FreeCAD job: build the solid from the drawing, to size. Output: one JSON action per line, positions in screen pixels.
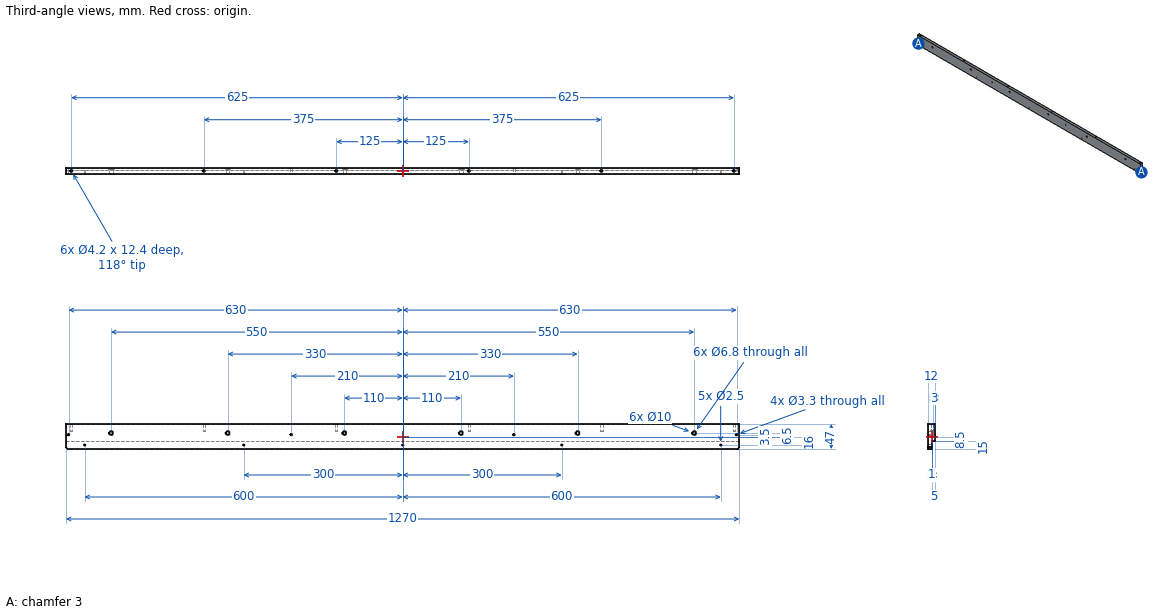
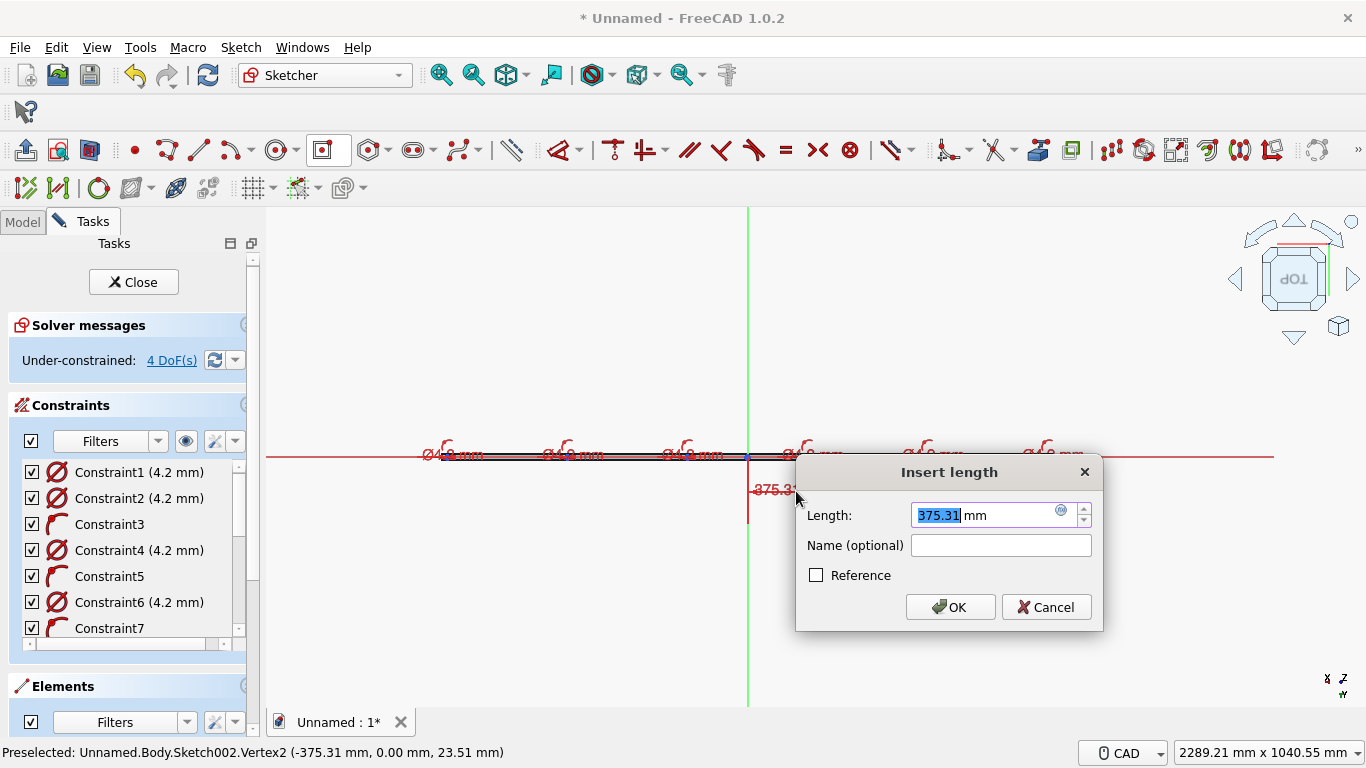
{"action": "type", "text": "375"}
{"action": "key", "text": "Return"}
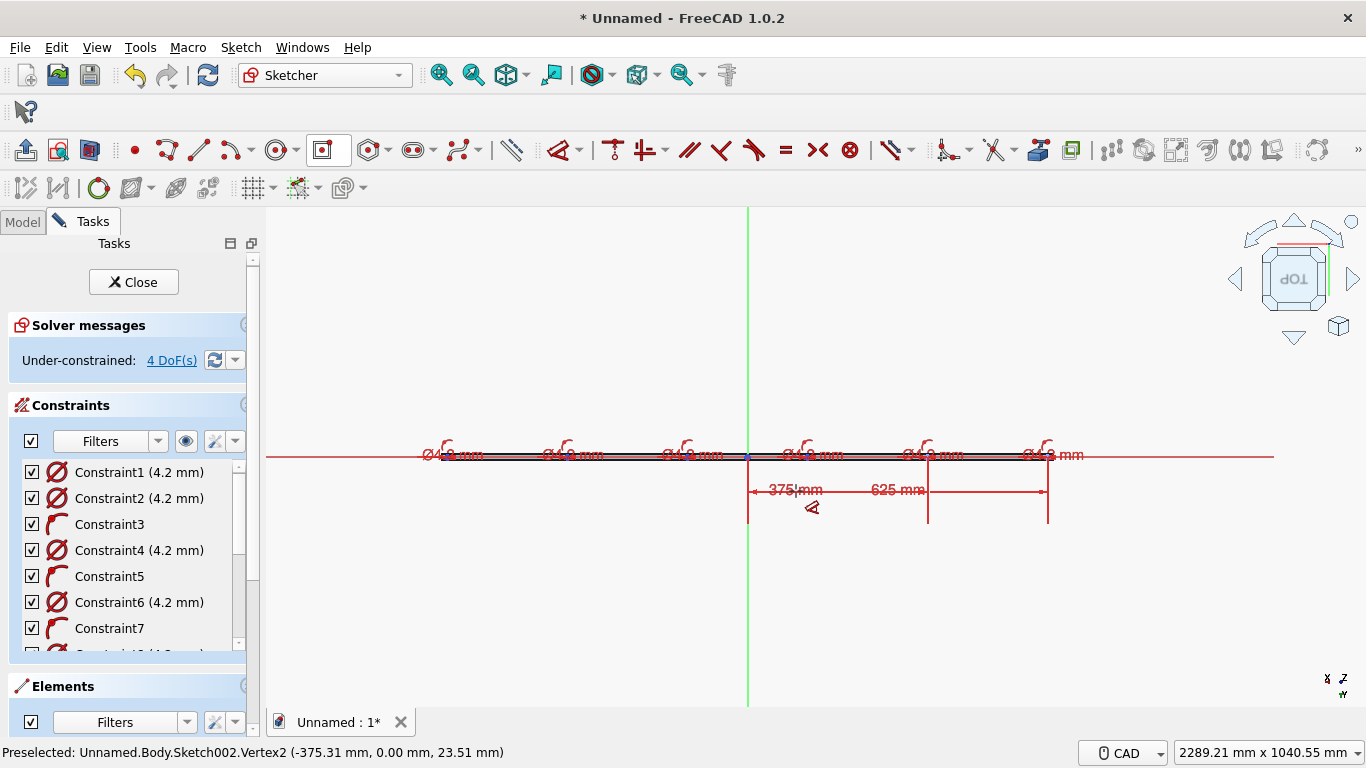
{"action": "left_click", "coordinate": [808, 457]}
{"action": "left_click", "coordinate": [778, 423]}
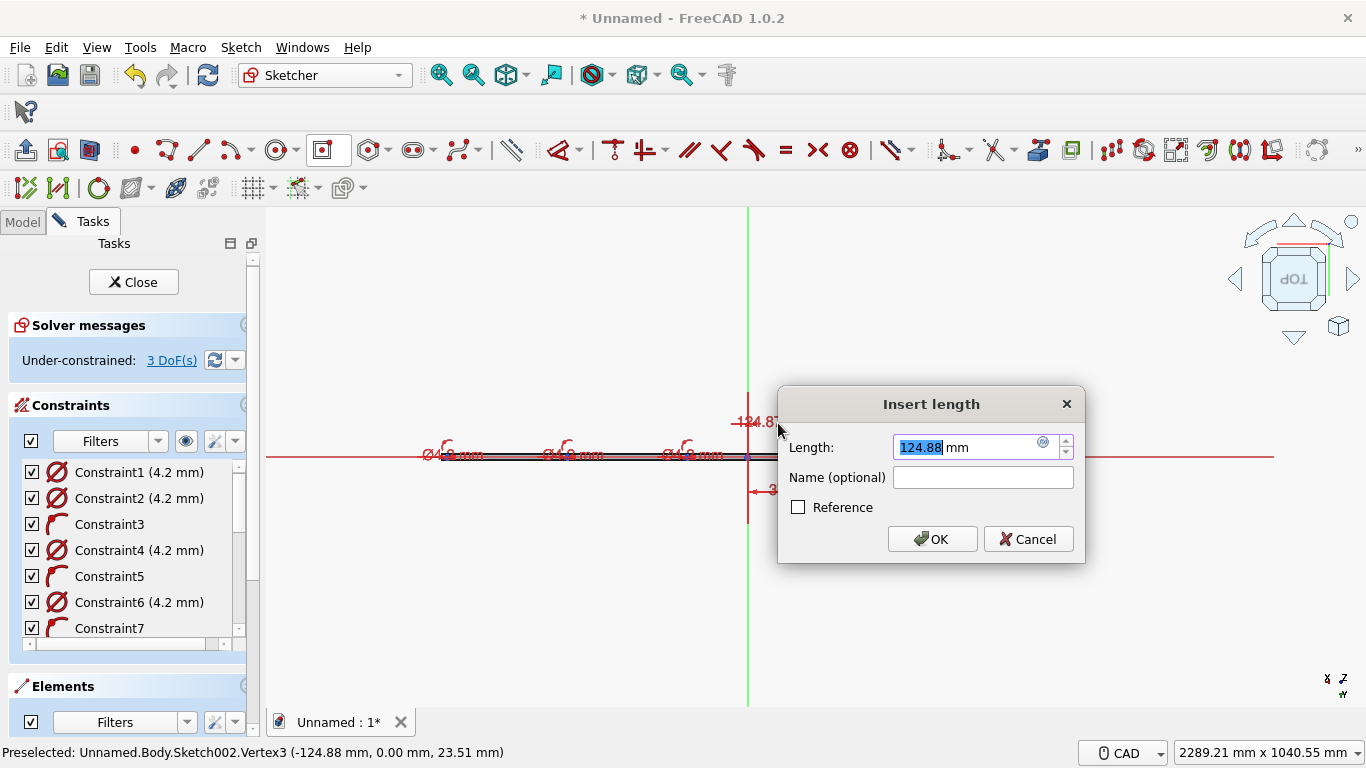
{"action": "type", "text": "125"}
{"action": "key", "text": "Return"}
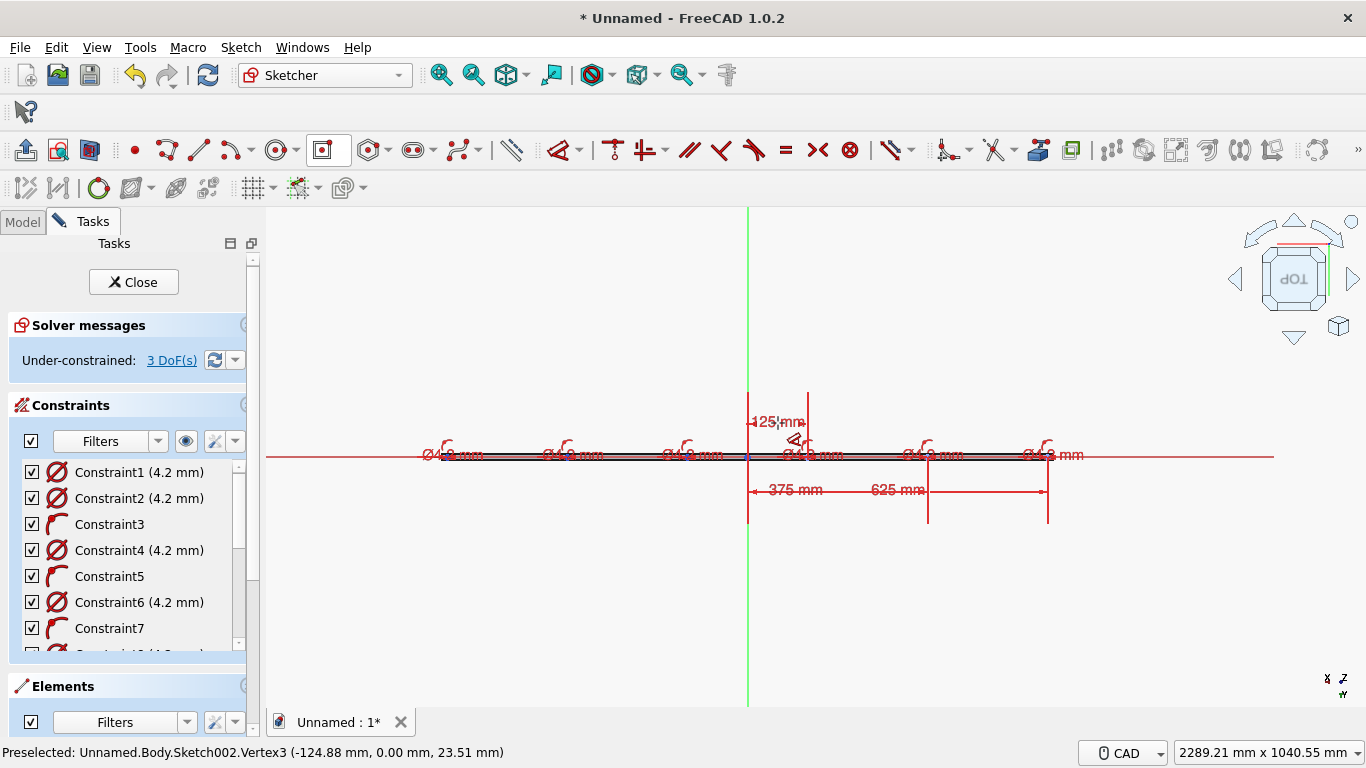
{"action": "left_click", "coordinate": [687, 457]}
{"action": "left_click", "coordinate": [717, 491]}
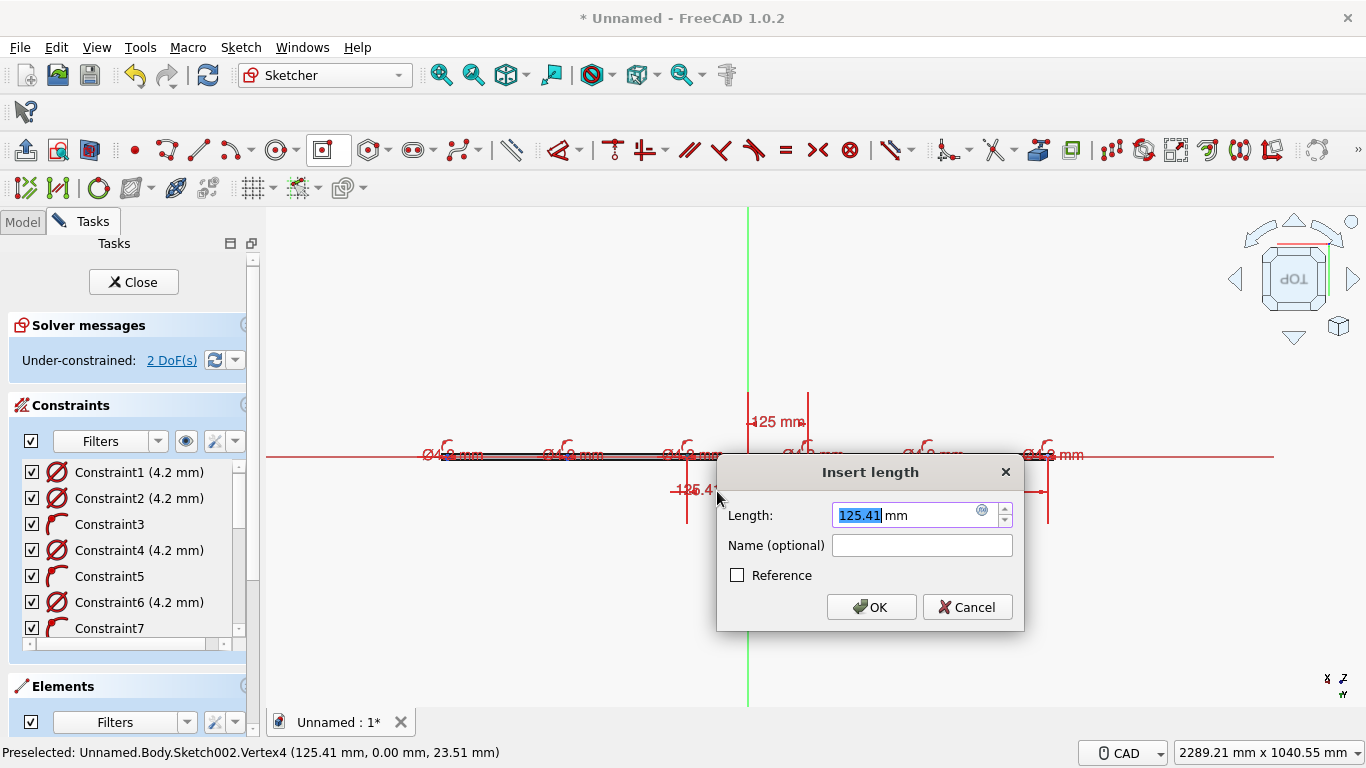
{"action": "type", "text": "125"}
{"action": "key", "text": "Return"}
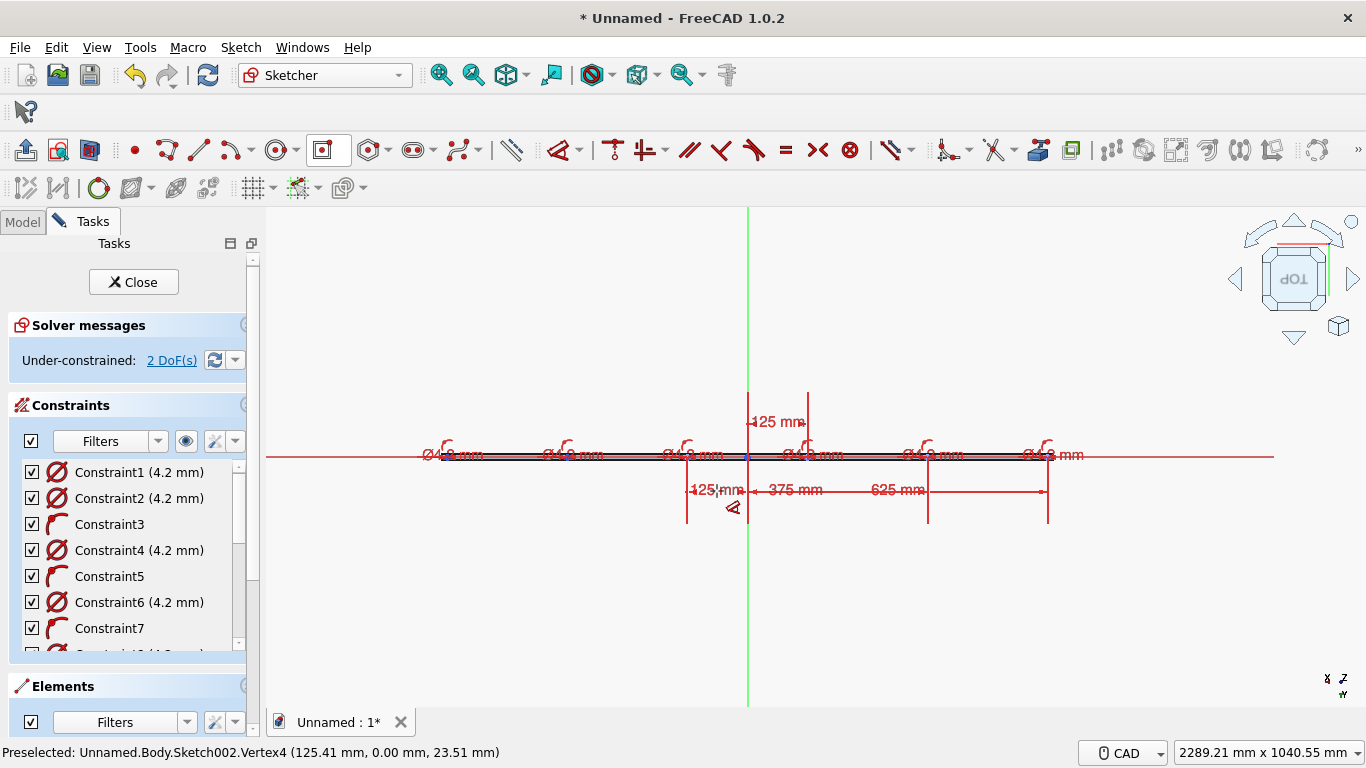
{"action": "left_click", "coordinate": [568, 457]}
{"action": "left_click", "coordinate": [616, 491]}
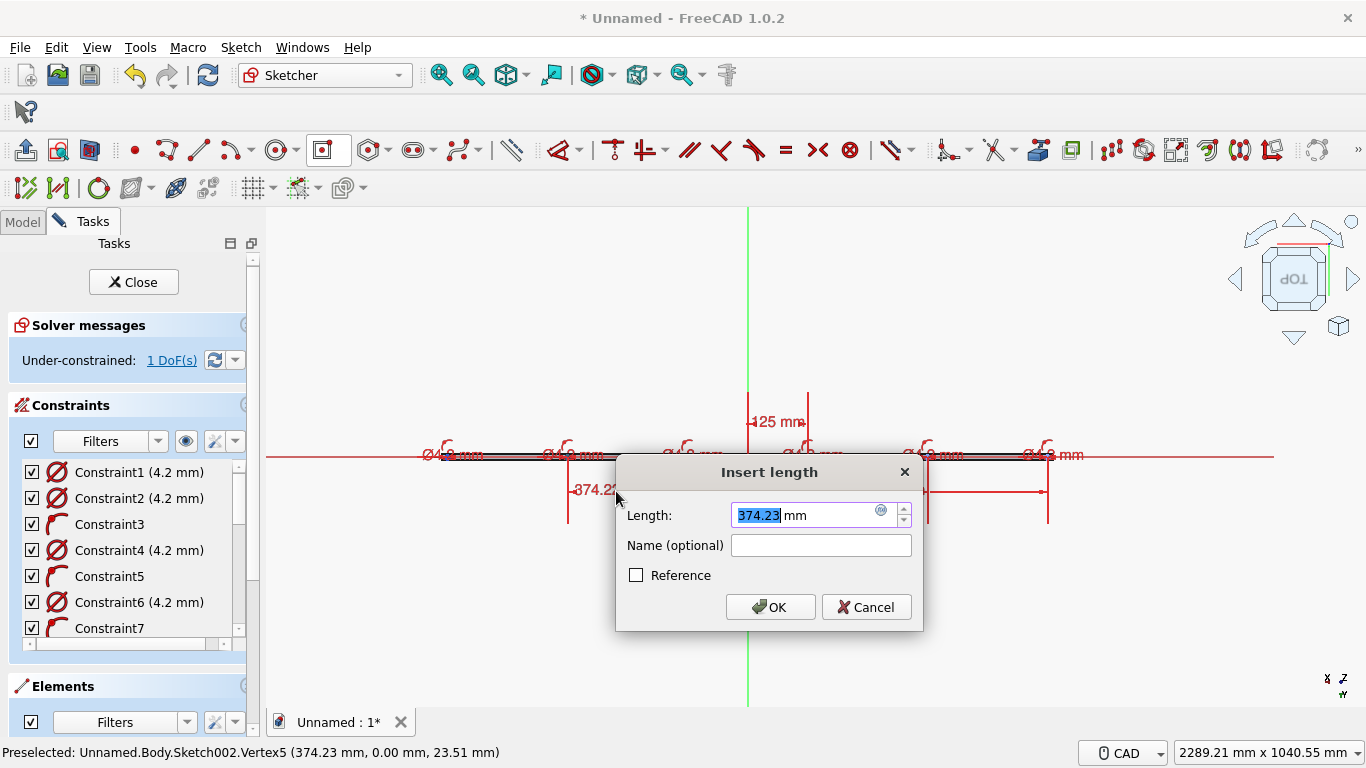
{"action": "type", "text": "375"}
{"action": "key", "text": "Return"}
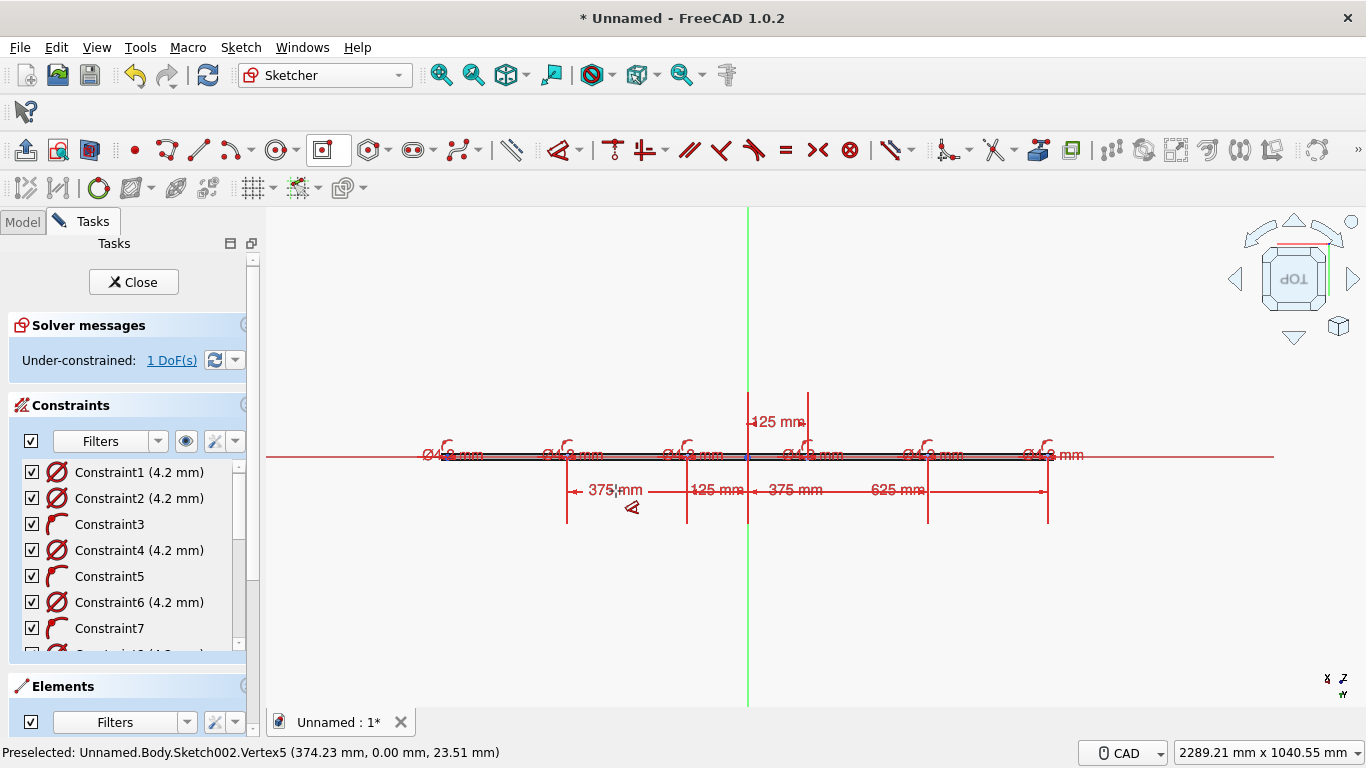
{"action": "left_click", "coordinate": [447, 457]}
{"action": "left_click", "coordinate": [528, 491]}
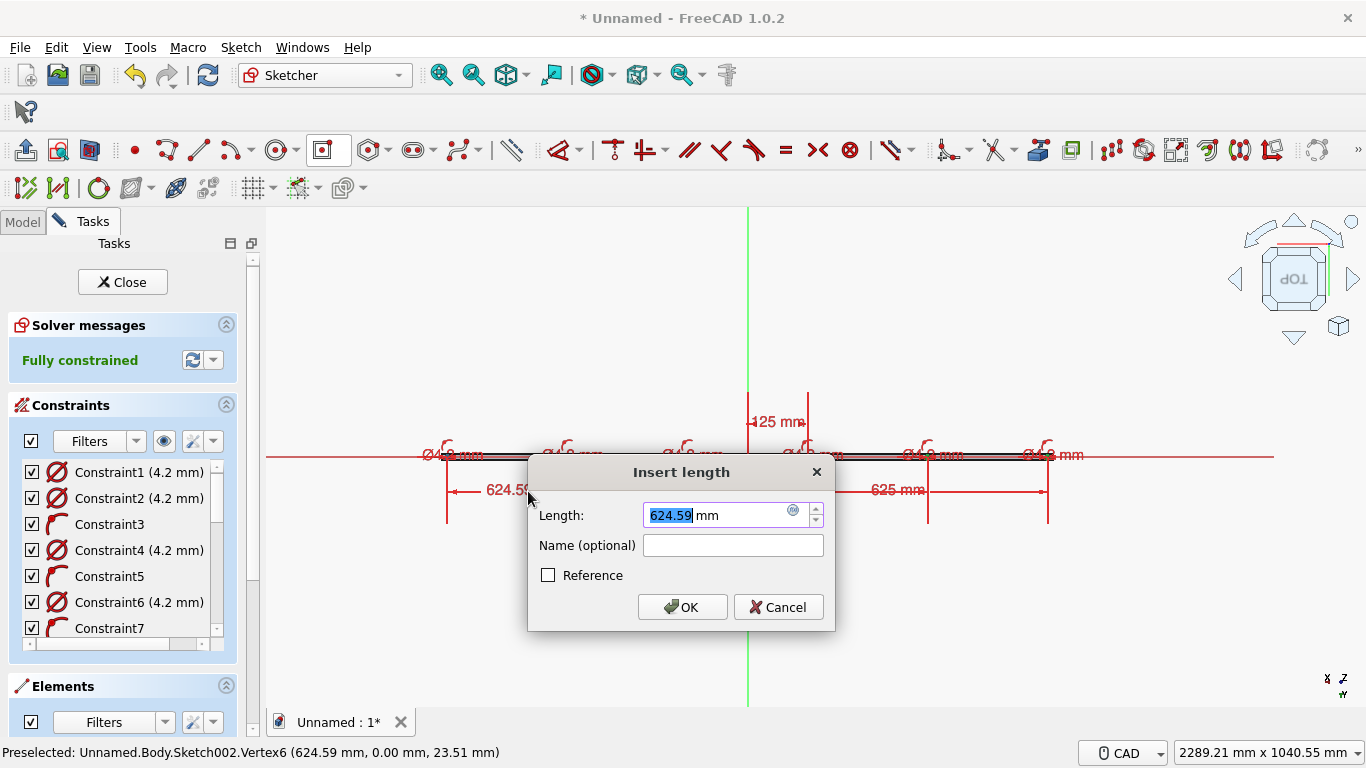
{"action": "type", "text": "625"}
{"action": "key", "text": "Return"}
{"action": "key", "text": "Escape"}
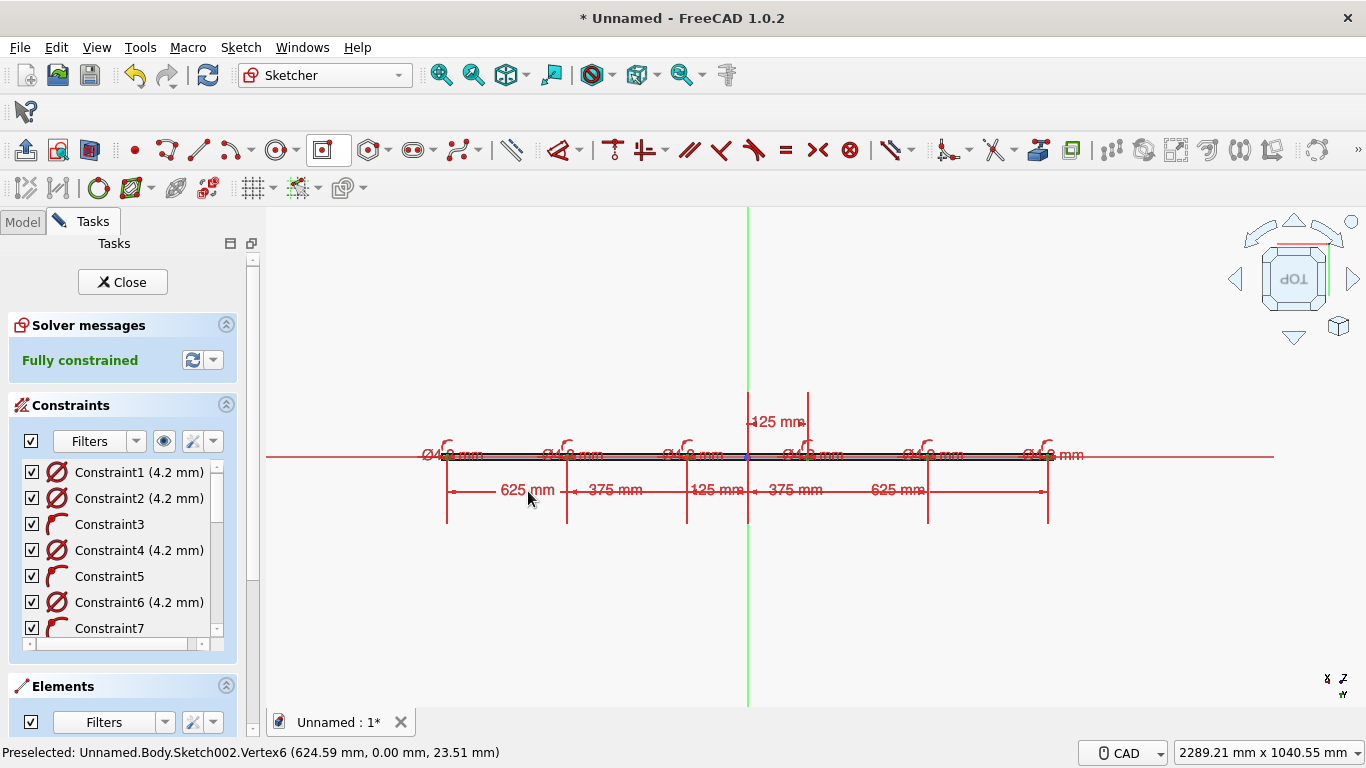
{"action": "left_click", "coordinate": [123, 282]}